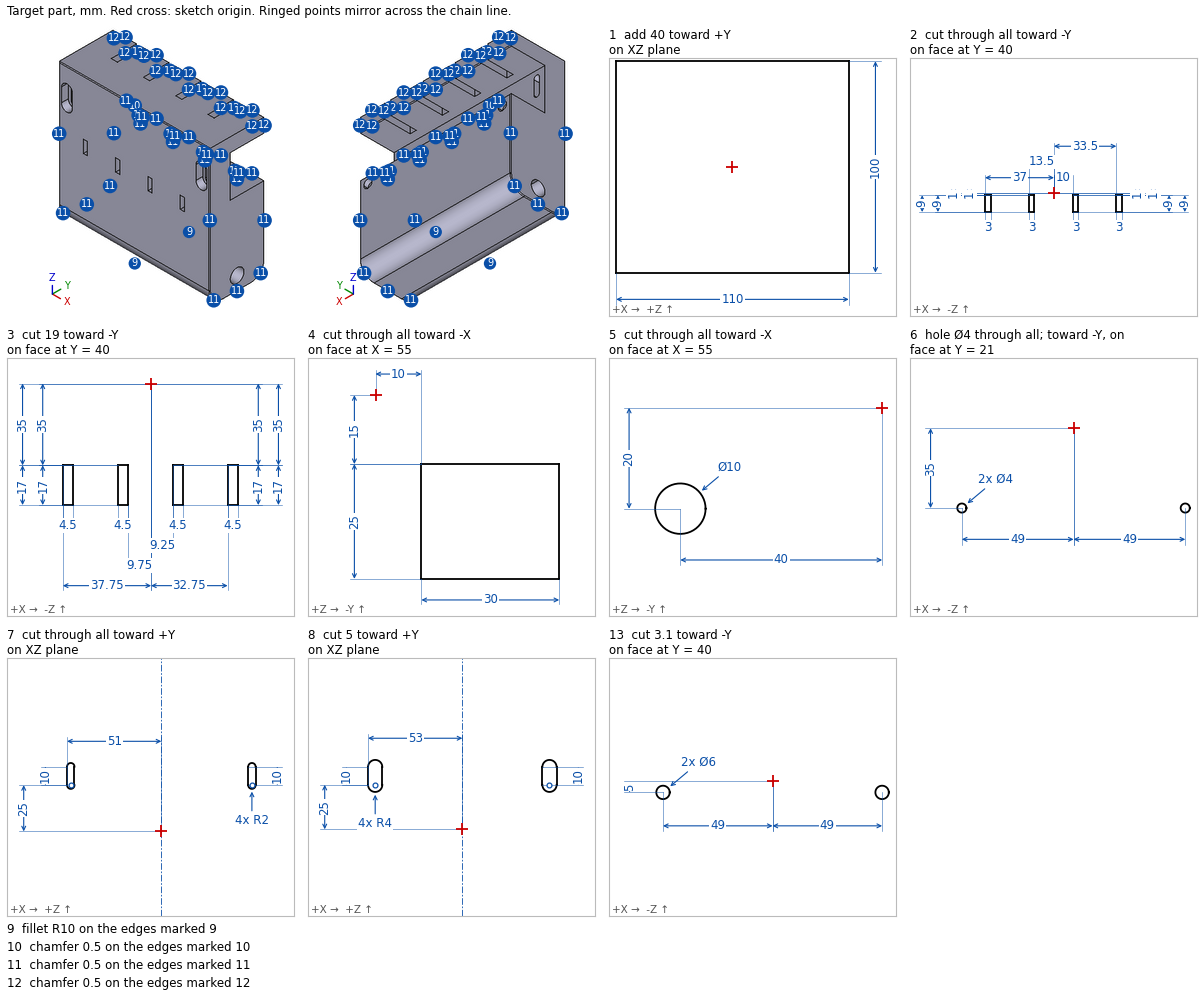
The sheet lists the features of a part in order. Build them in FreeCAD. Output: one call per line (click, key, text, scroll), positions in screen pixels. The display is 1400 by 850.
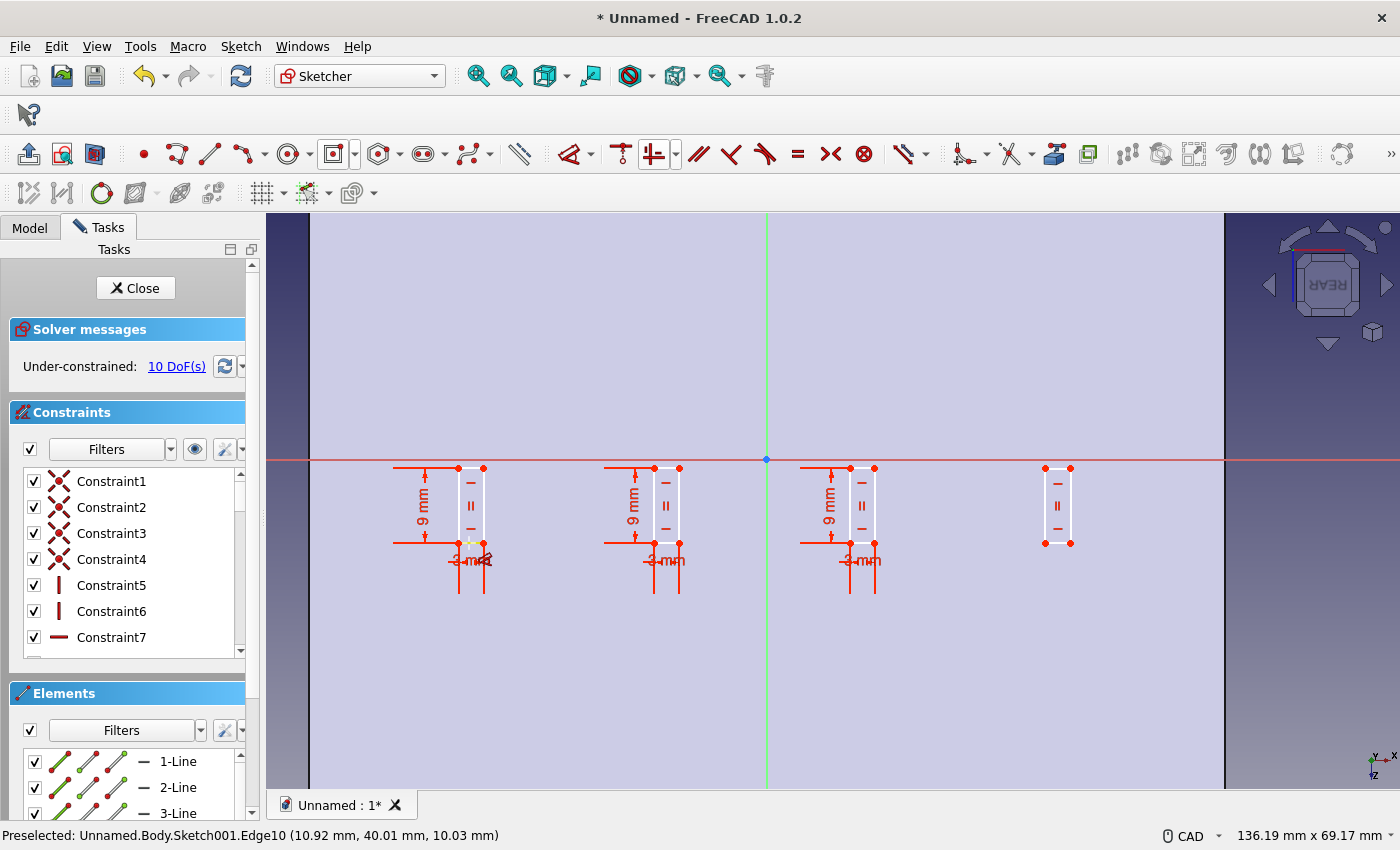
click(1045, 491)
click(1011, 506)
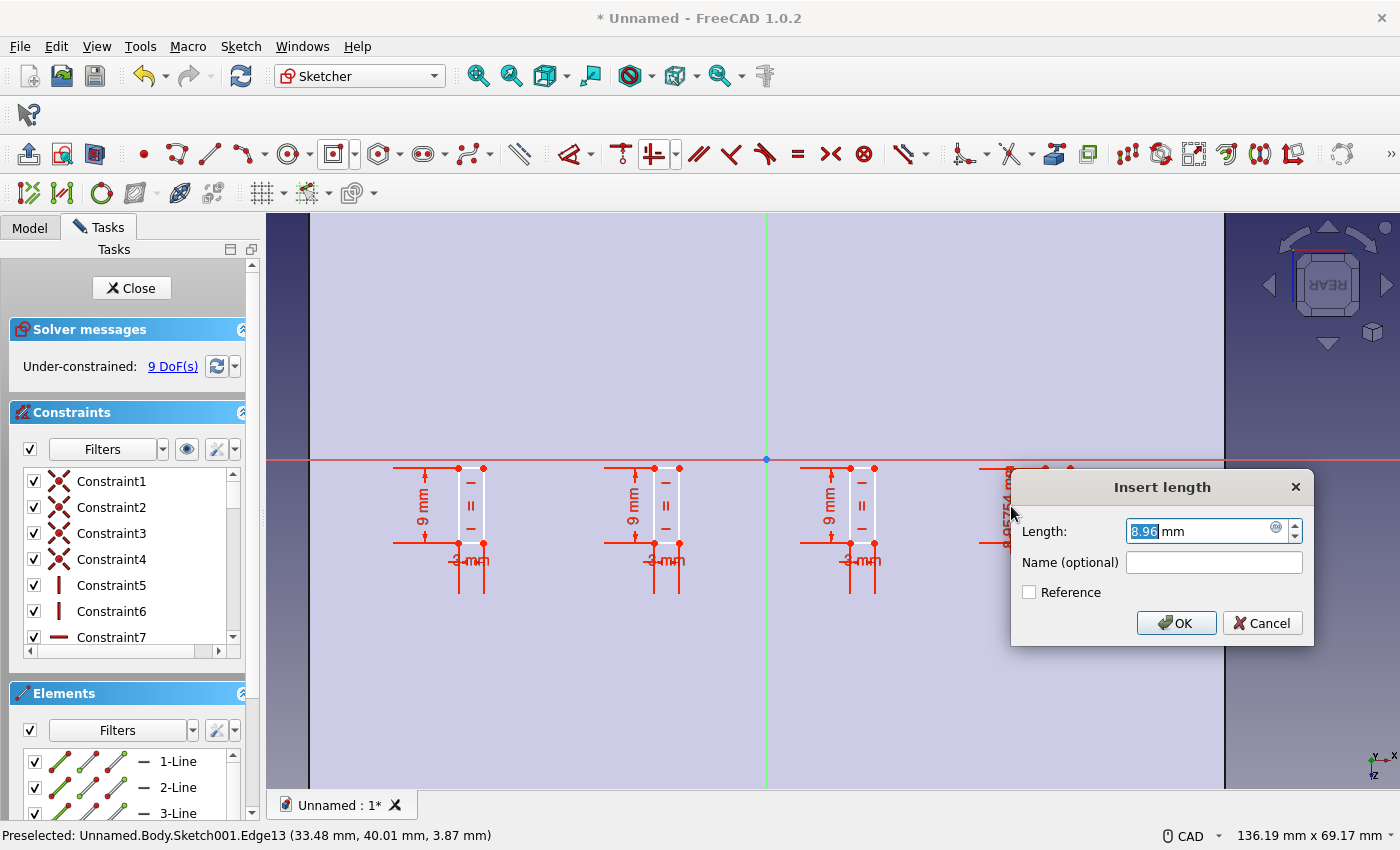
text(9)
key(Return)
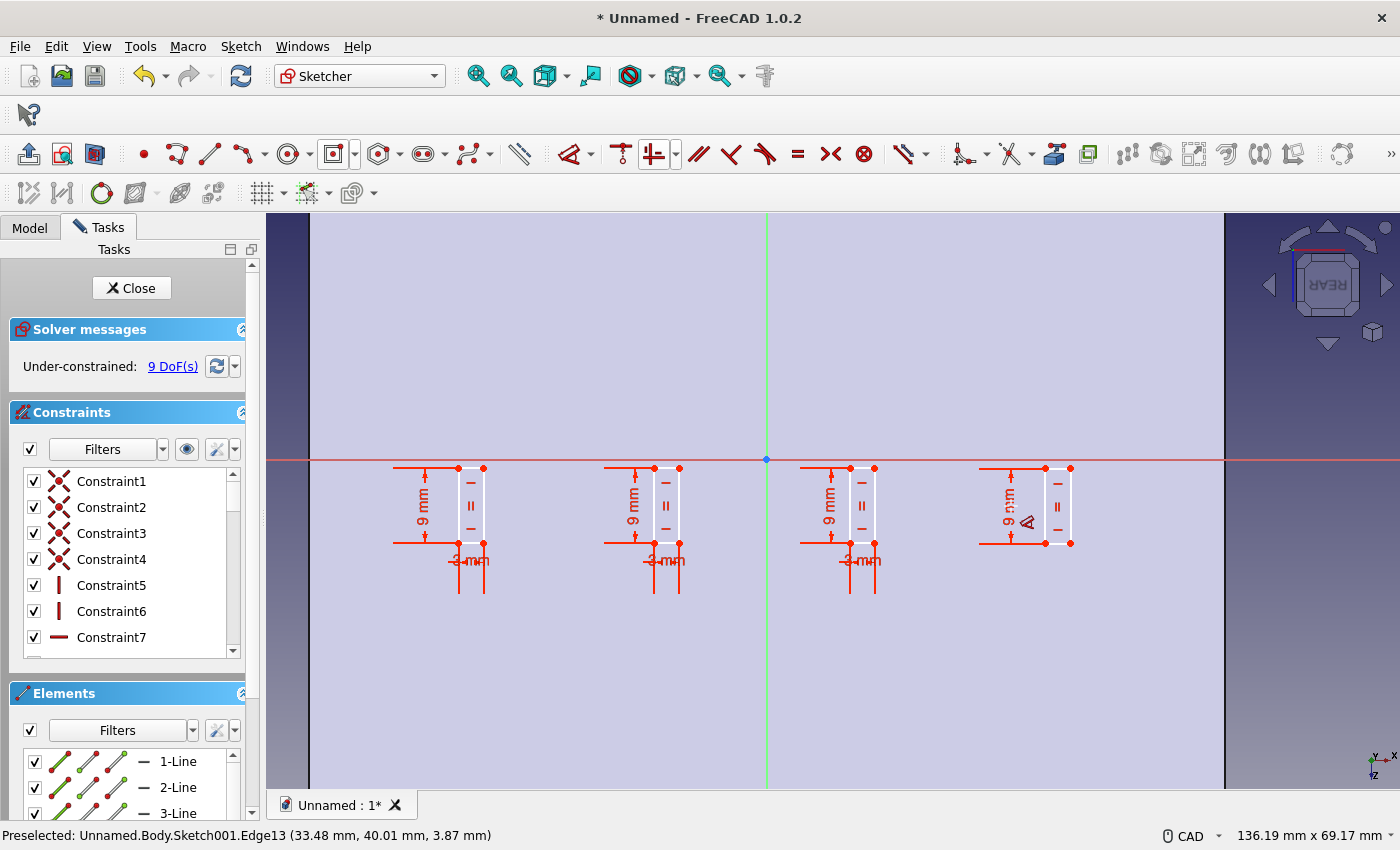
scroll(1056, 544, up, 3)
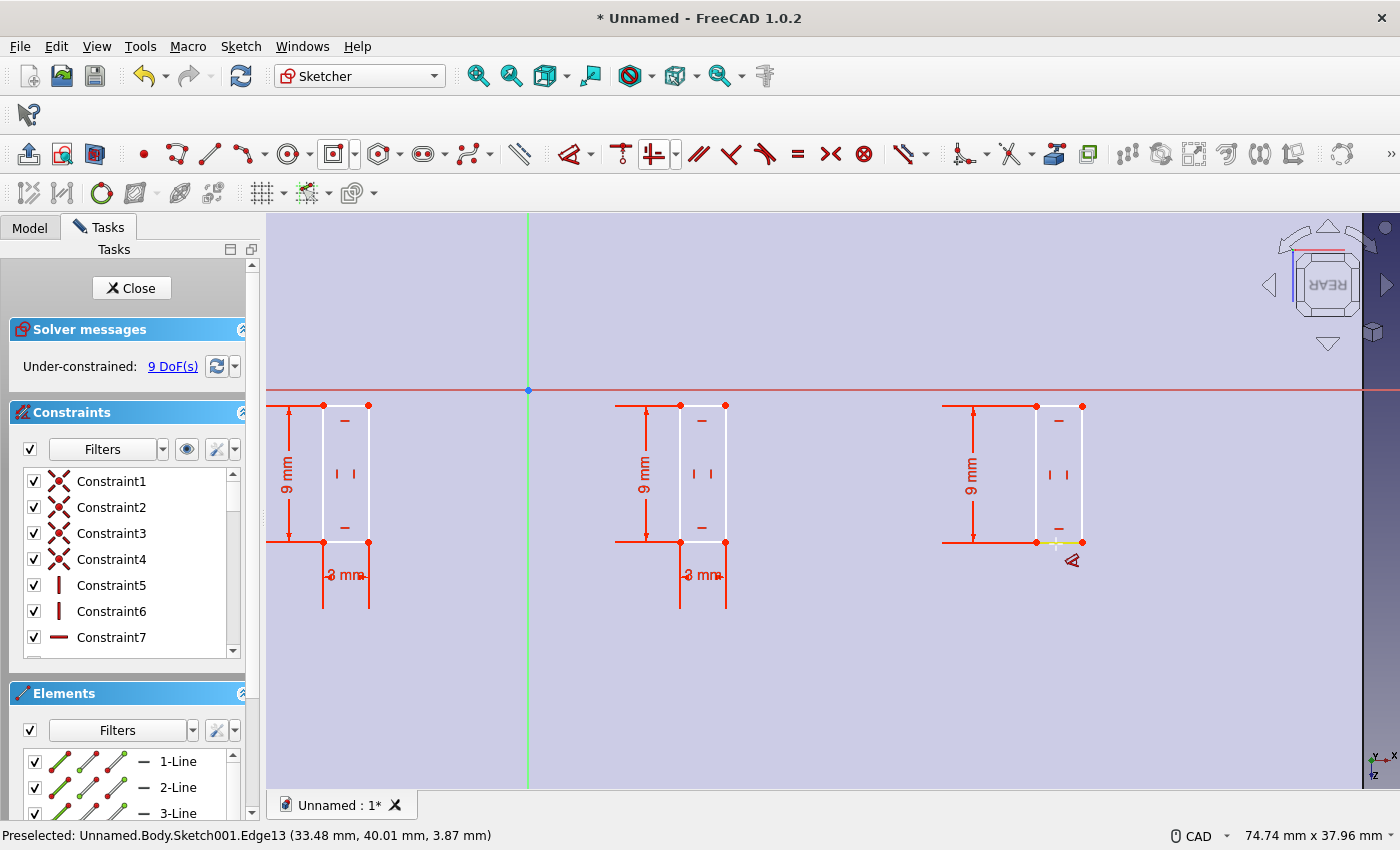
click(1055, 543)
click(1059, 577)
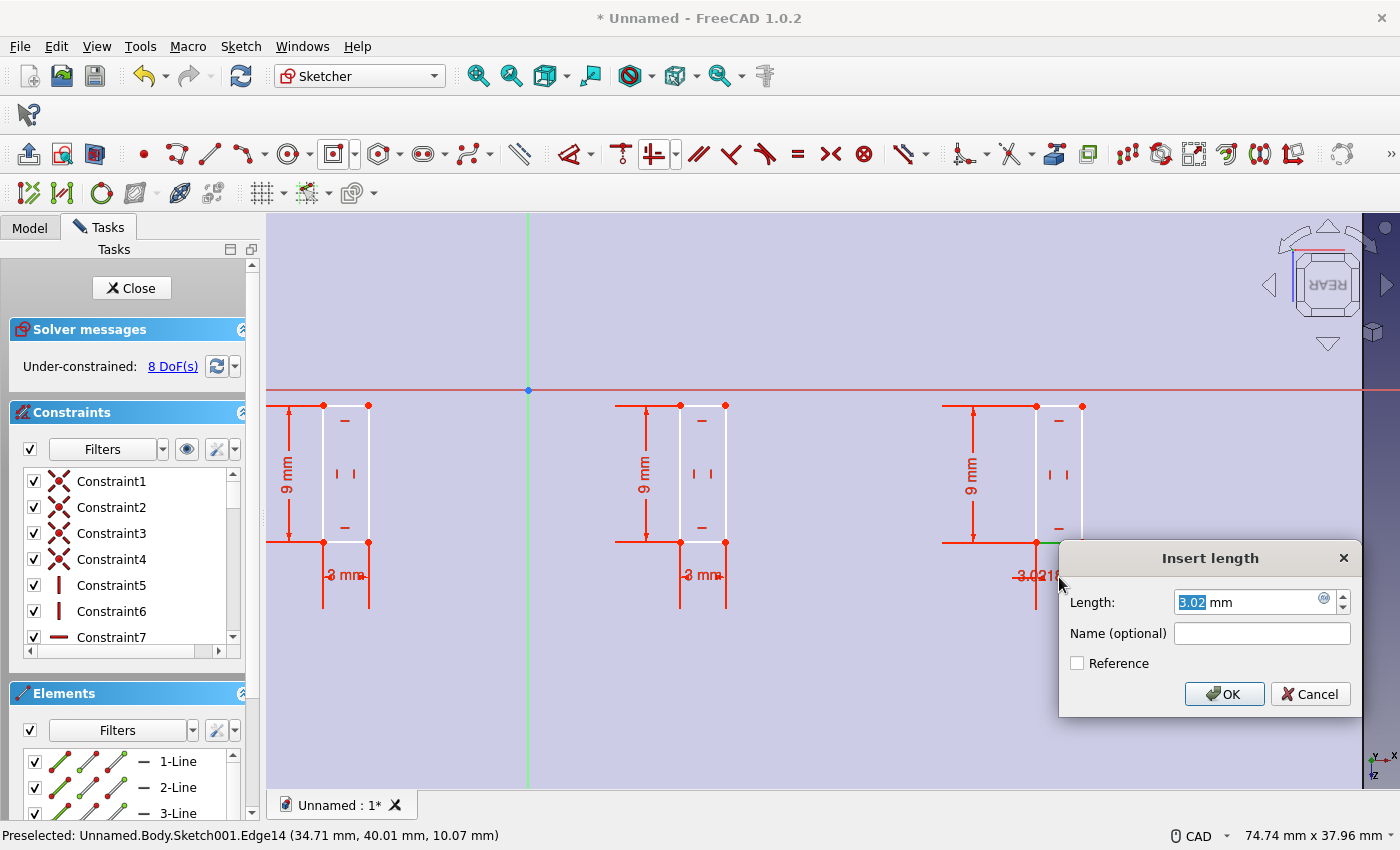
text(3)
key(Return)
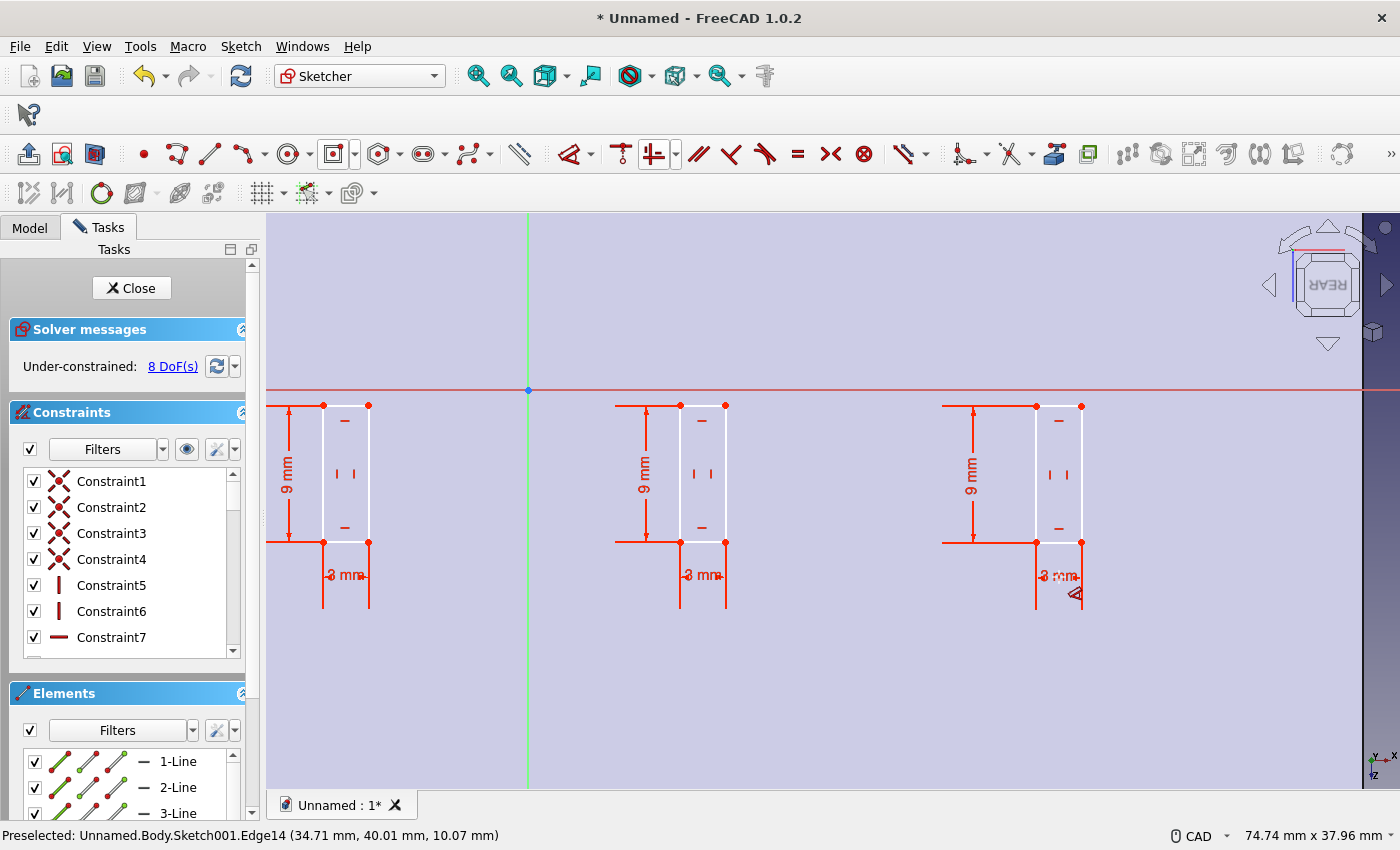
scroll(1056, 544, down, 3)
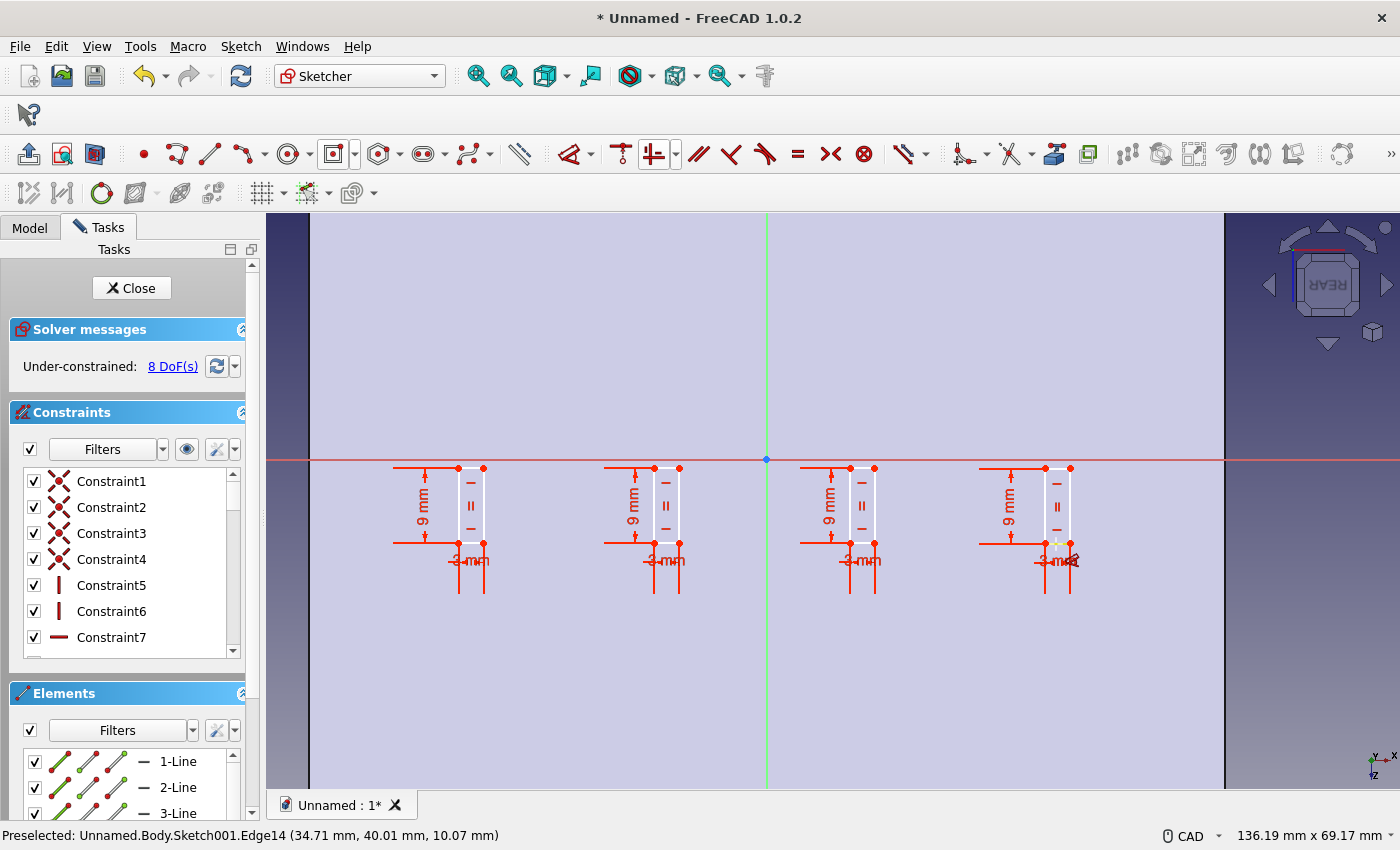
scroll(459, 468, up, 8)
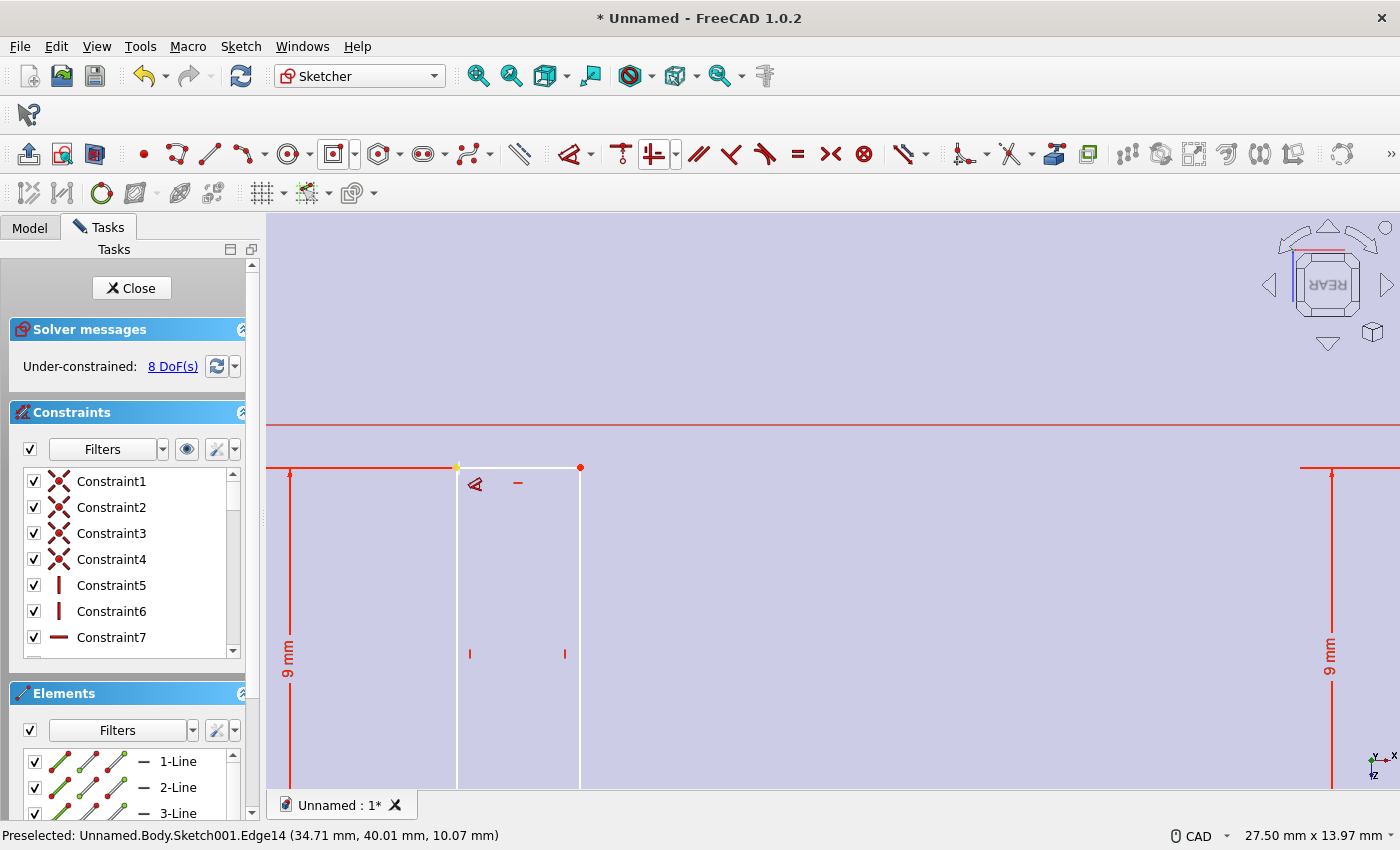
click(457, 468)
click(423, 447)